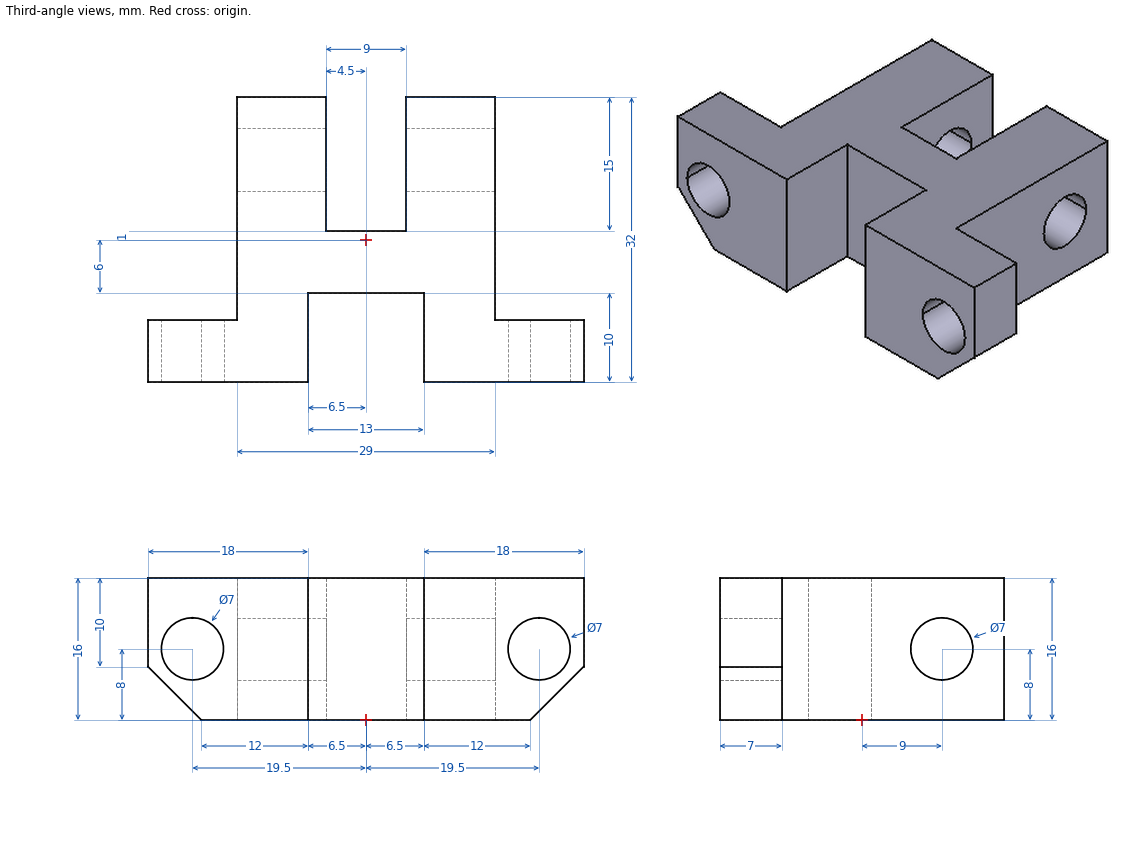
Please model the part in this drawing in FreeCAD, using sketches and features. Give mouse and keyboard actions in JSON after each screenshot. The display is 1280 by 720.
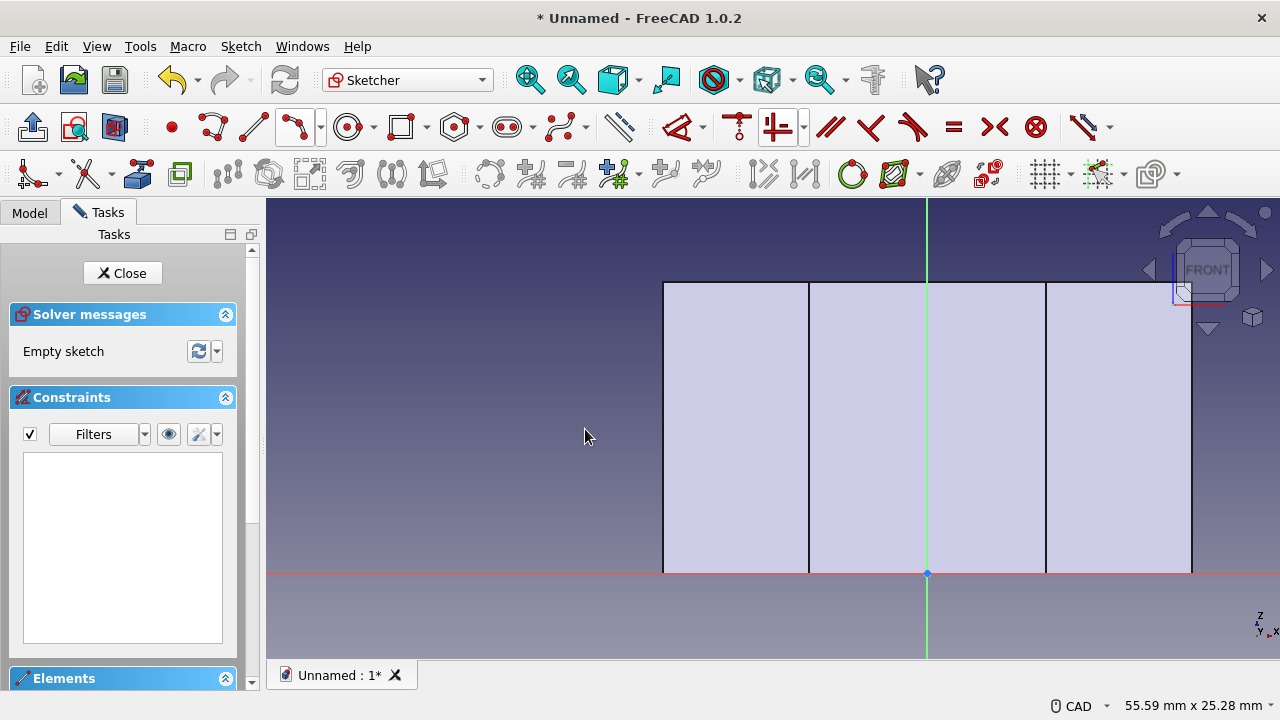
{"action": "left_click", "coordinate": [213, 128]}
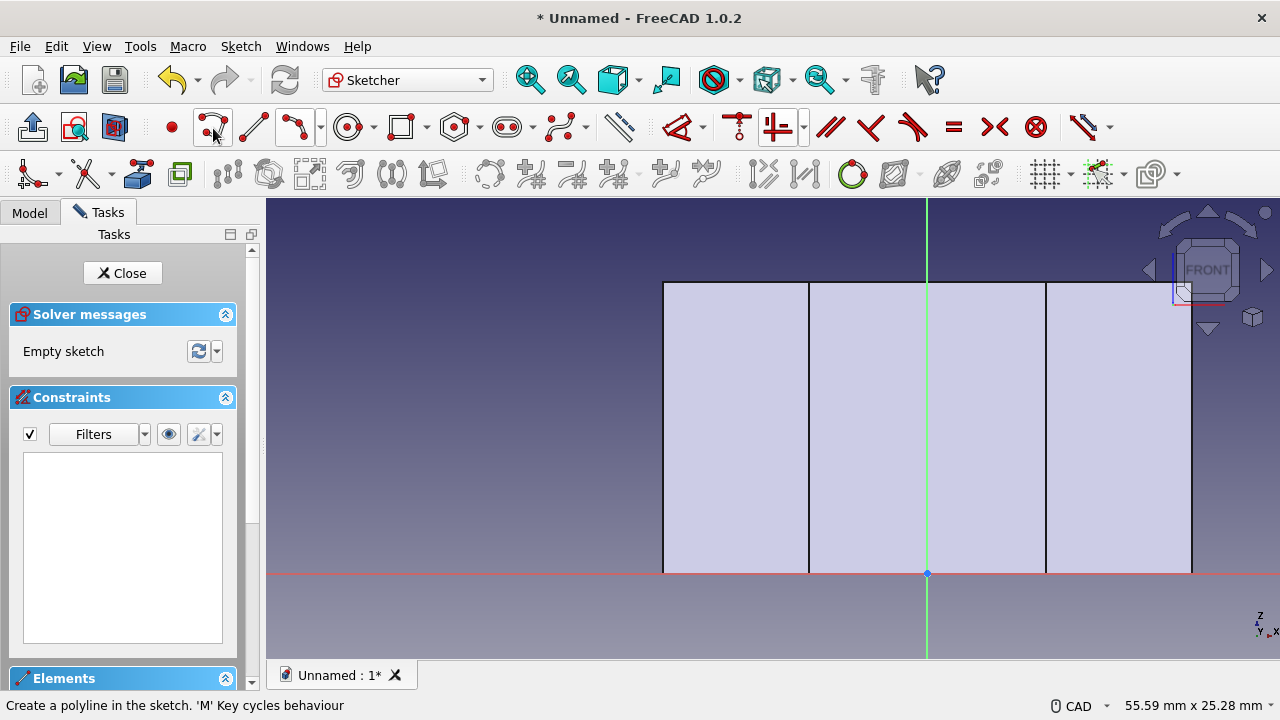
{"action": "left_click", "coordinate": [809, 574]}
{"action": "left_click", "coordinate": [809, 282]}
{"action": "left_click", "coordinate": [480, 282]}
{"action": "left_click", "coordinate": [480, 464]}
{"action": "left_click", "coordinate": [590, 565]}
{"action": "left_click", "coordinate": [809, 574]}
{"action": "key", "text": "Escape"}
{"action": "key", "text": "Escape"}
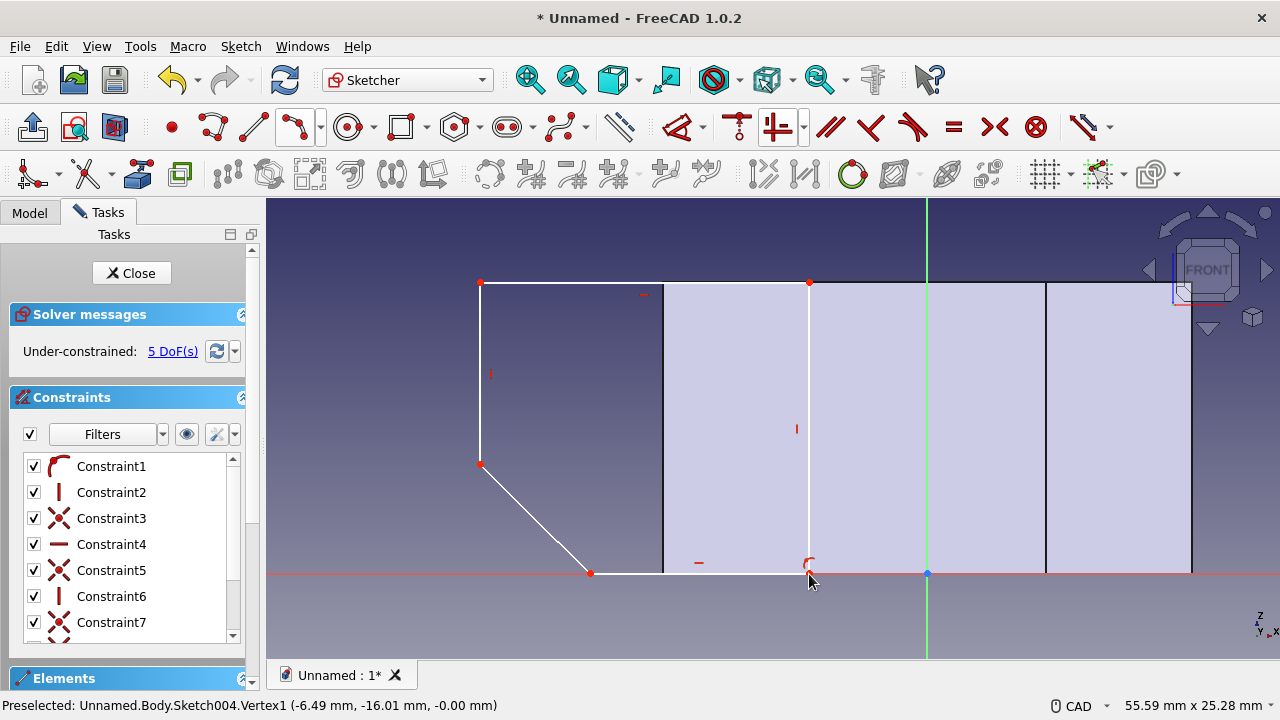
{"action": "left_click", "coordinate": [676, 128]}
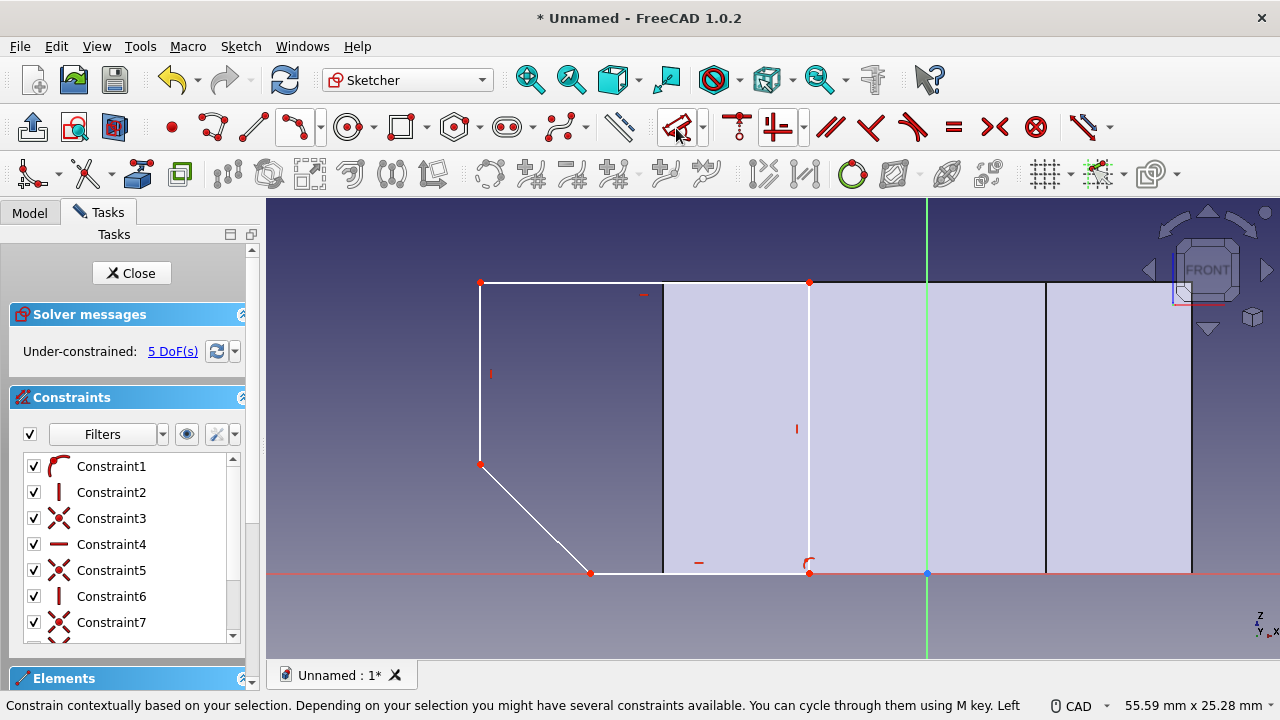
{"action": "left_click", "coordinate": [809, 486]}
{"action": "left_click", "coordinate": [843, 428]}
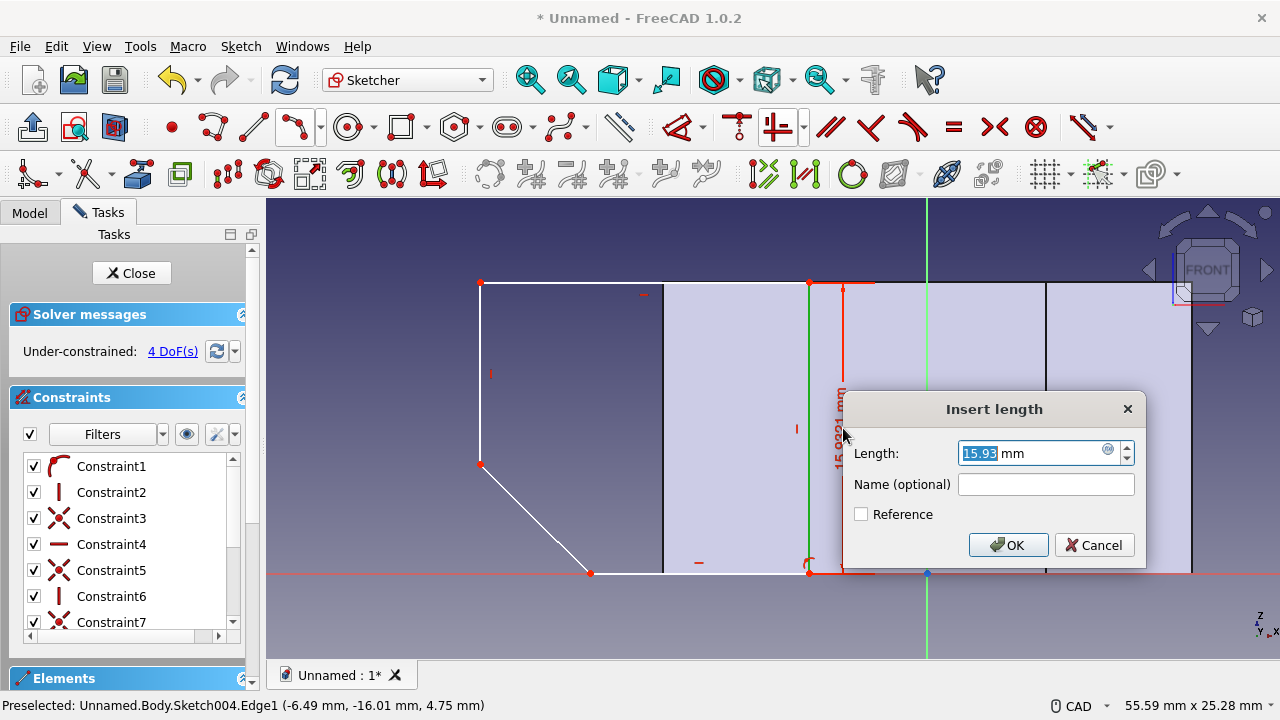
{"action": "type", "text": "16"}
{"action": "key", "text": "Return"}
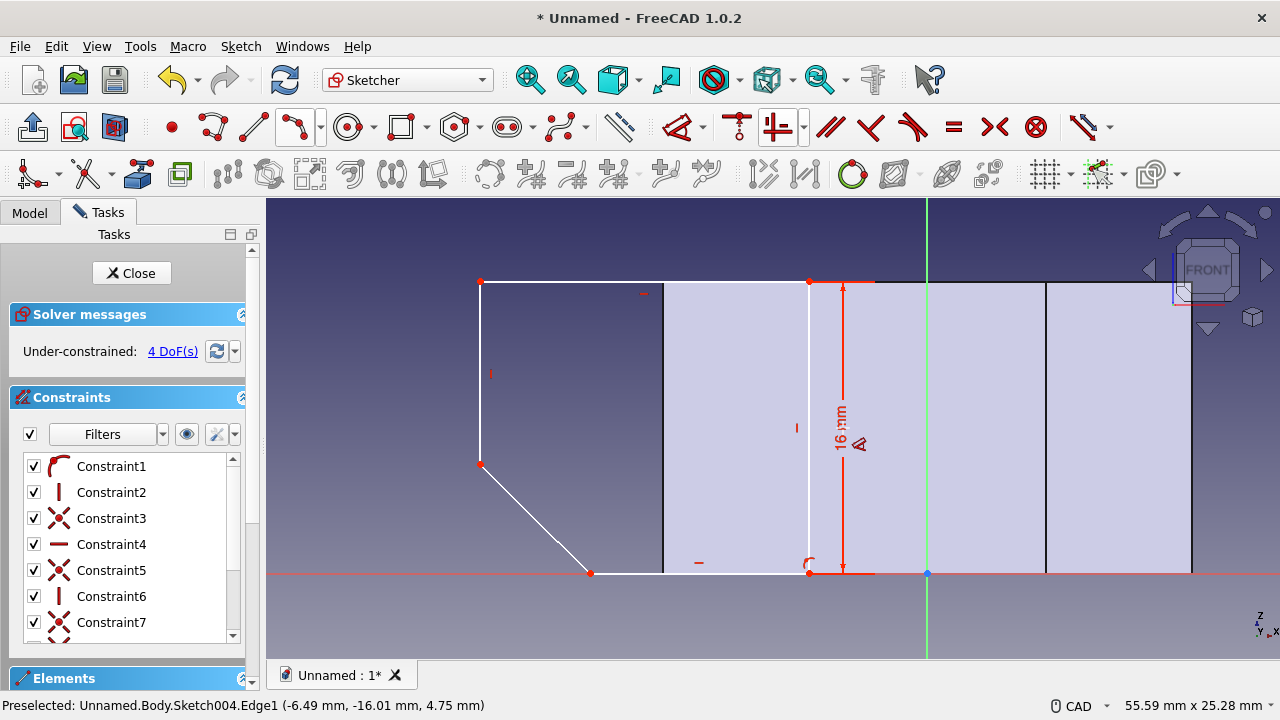
{"action": "left_click", "coordinate": [710, 282]}
{"action": "left_click", "coordinate": [645, 248]}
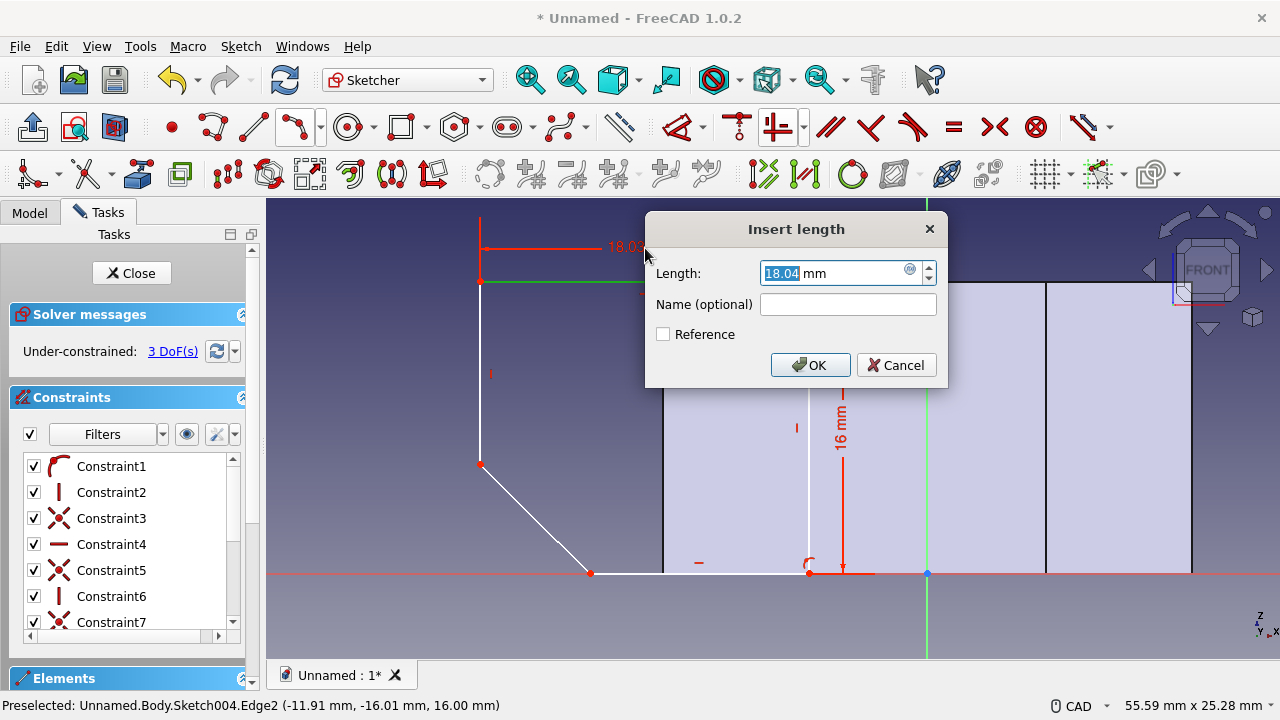
{"action": "type", "text": "18"}
{"action": "key", "text": "Return"}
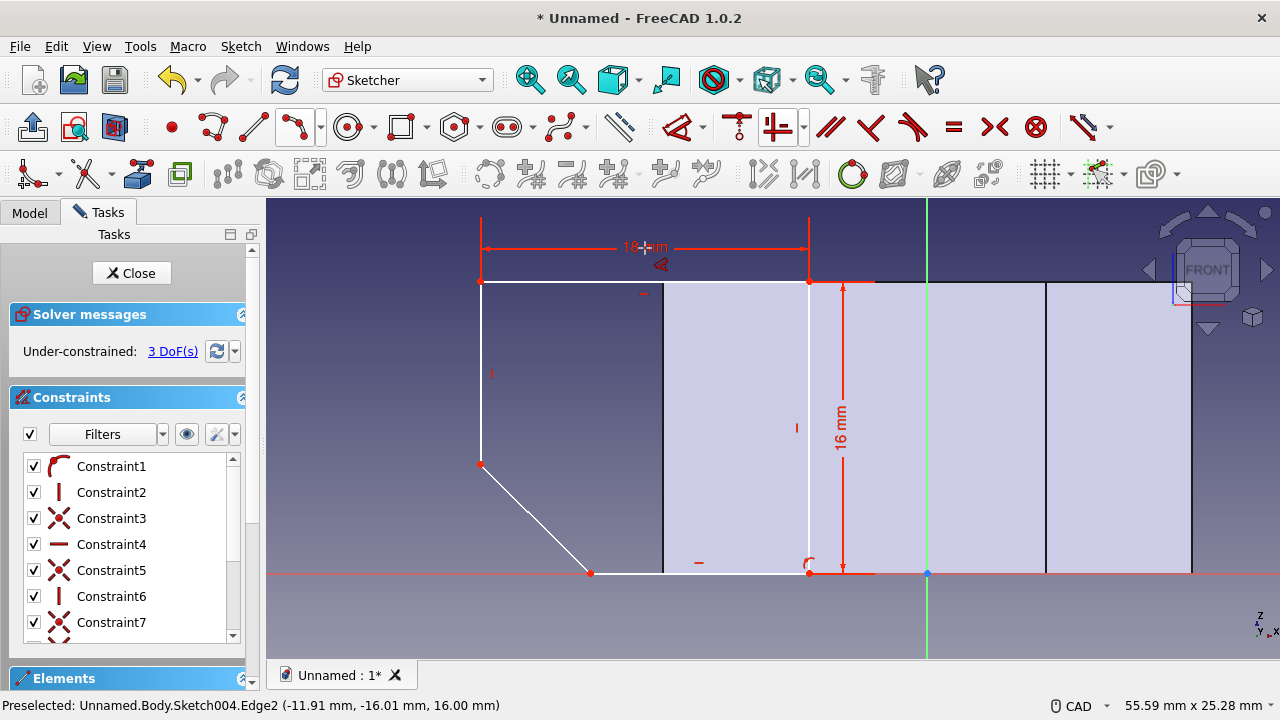
{"action": "left_click", "coordinate": [481, 337]}
{"action": "left_click", "coordinate": [447, 373]}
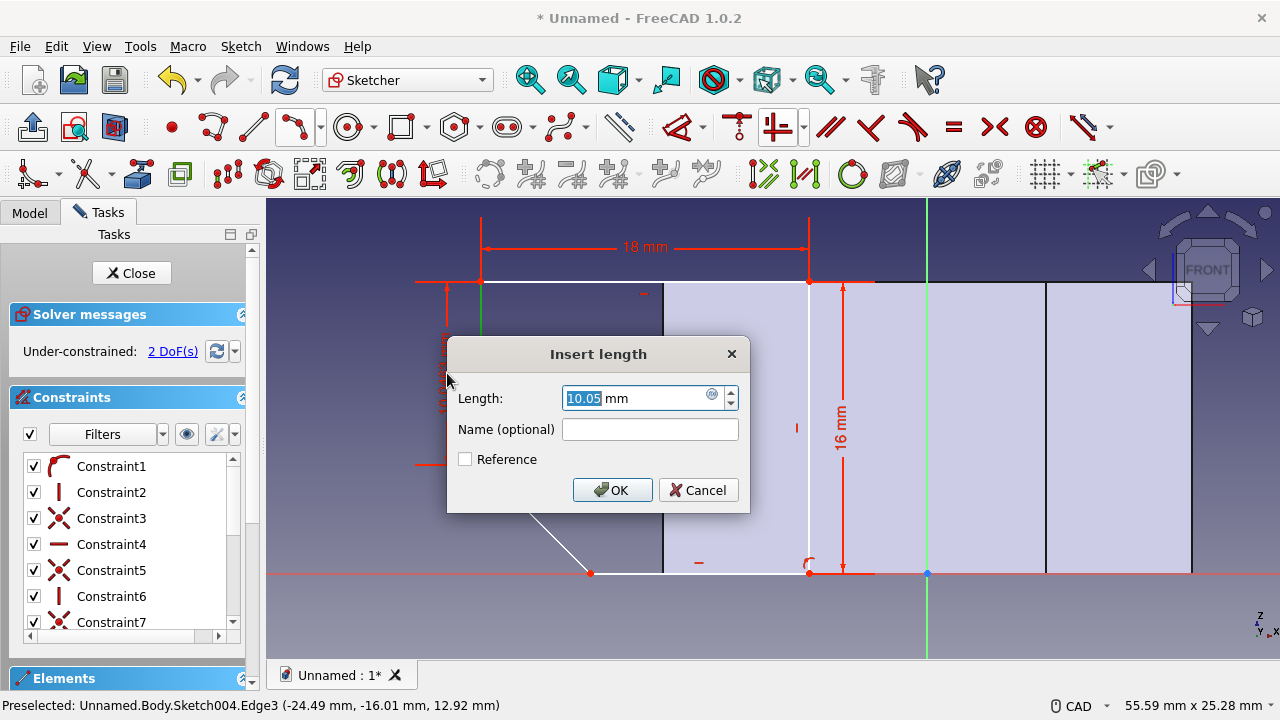
{"action": "type", "text": "10"}
{"action": "key", "text": "Return"}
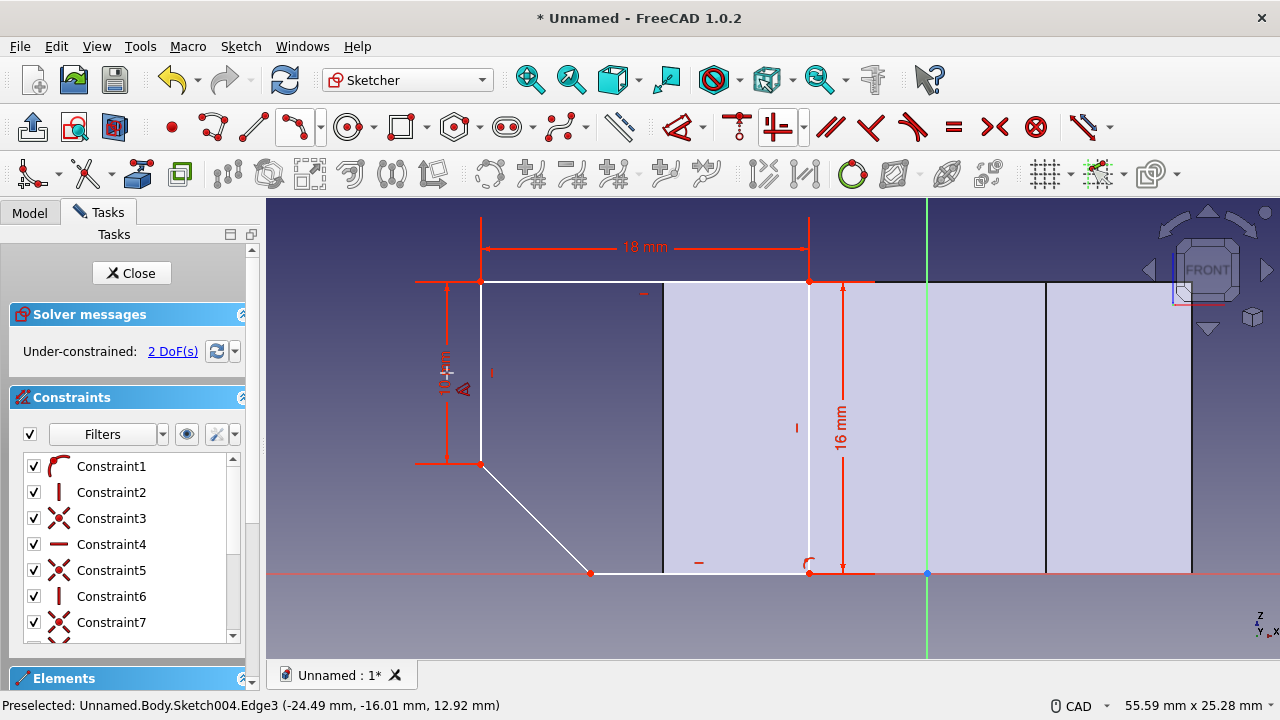
{"action": "left_click", "coordinate": [656, 574]}
{"action": "left_click", "coordinate": [699, 608]}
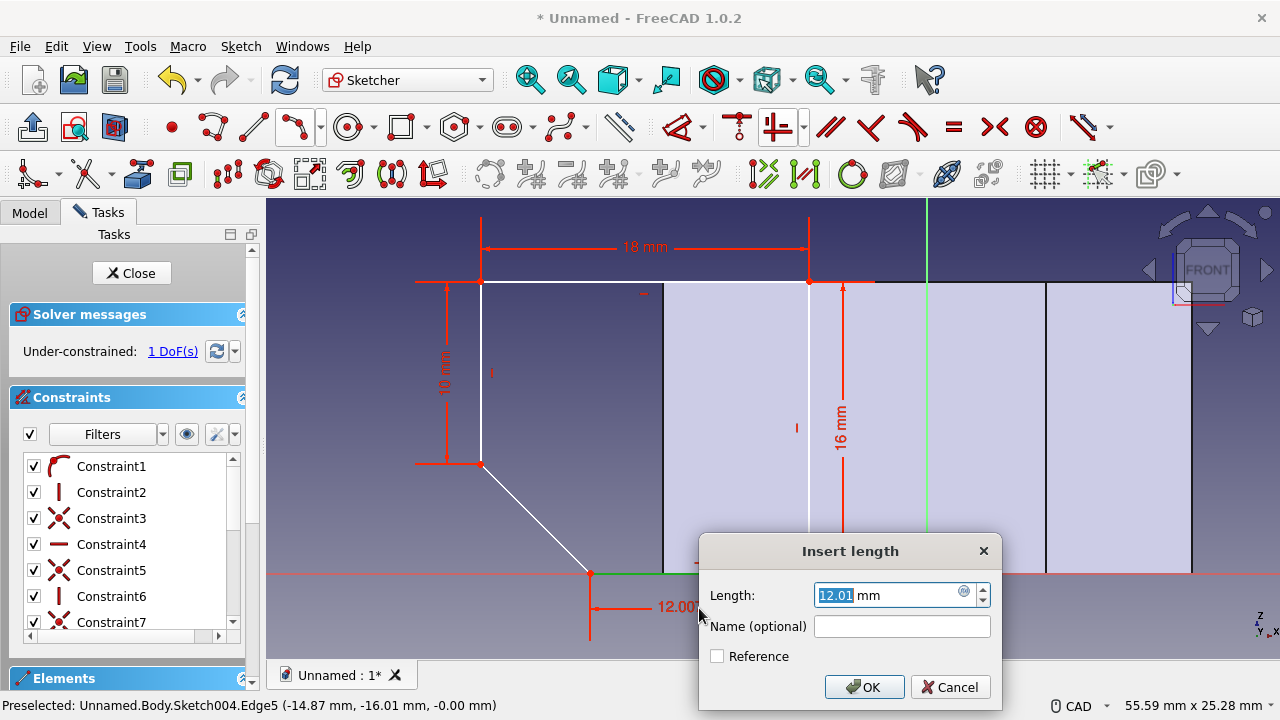
{"action": "type", "text": "12"}
{"action": "key", "text": "Return"}